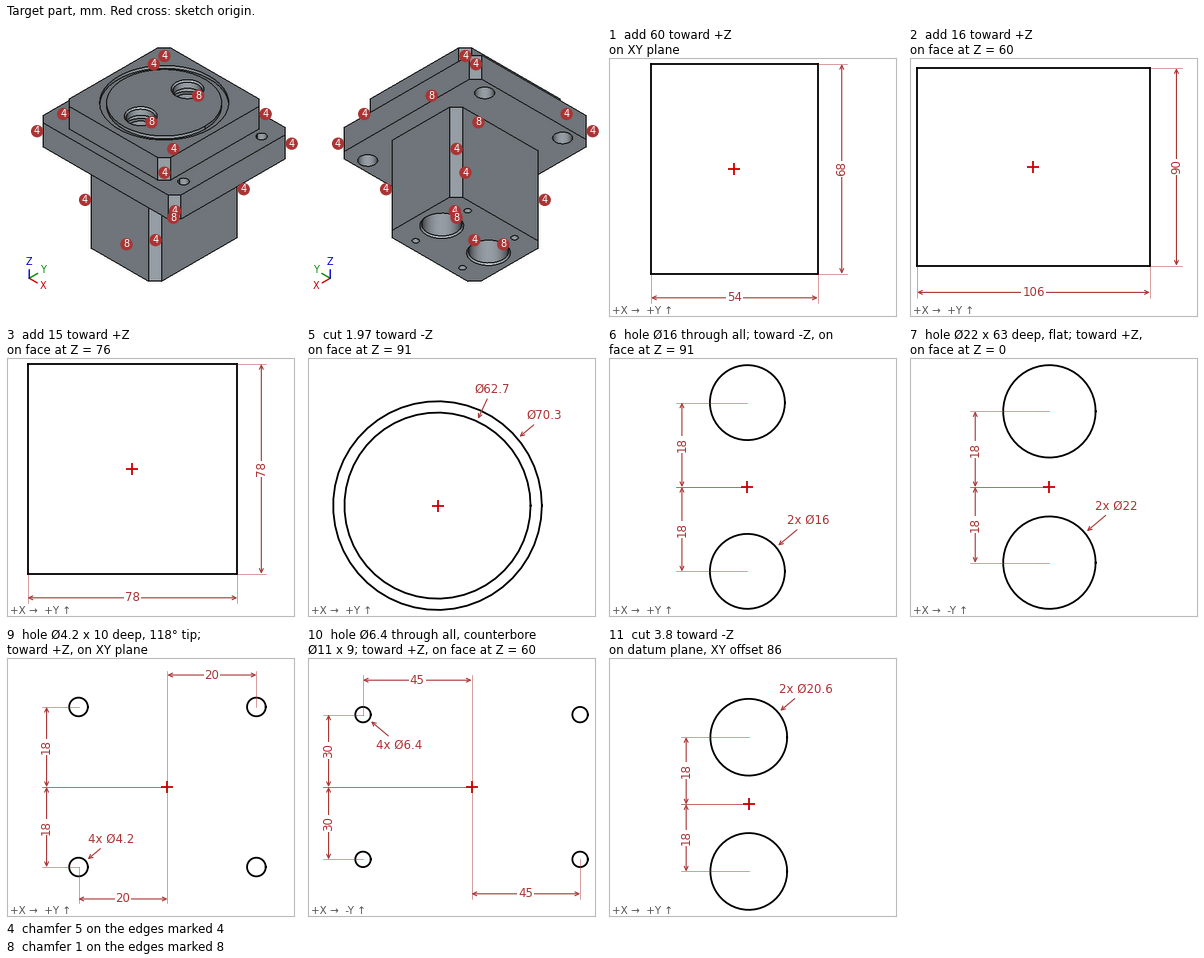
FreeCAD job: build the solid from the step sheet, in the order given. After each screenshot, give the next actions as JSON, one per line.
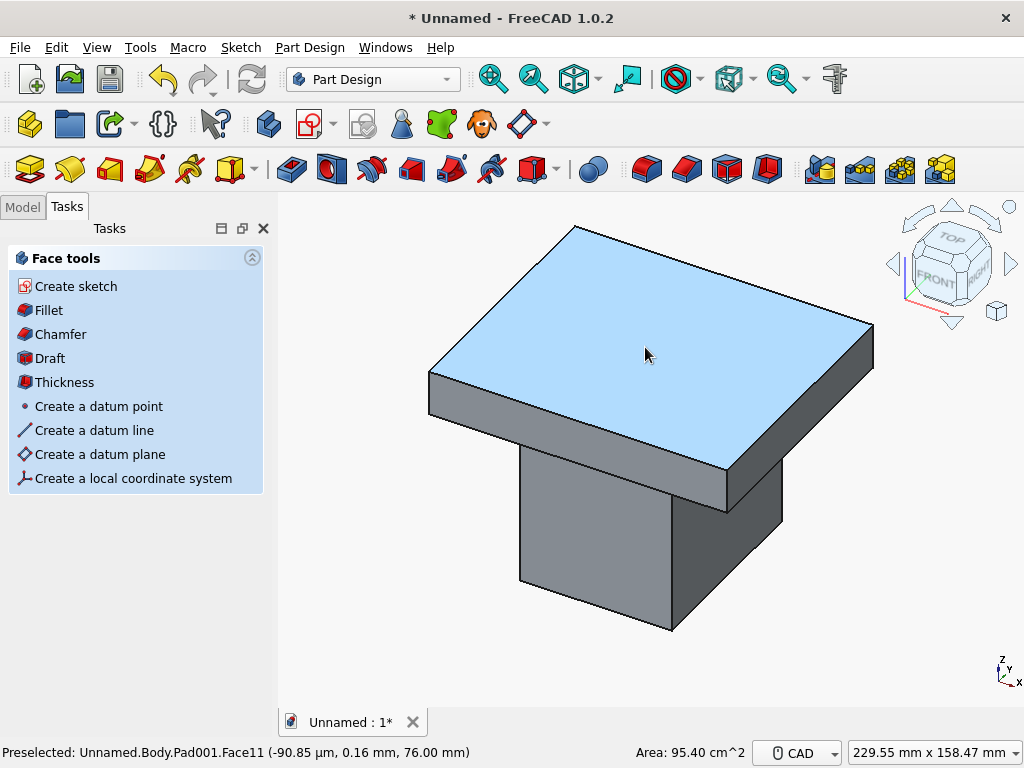
{"action": "left_click", "coordinate": [310, 124]}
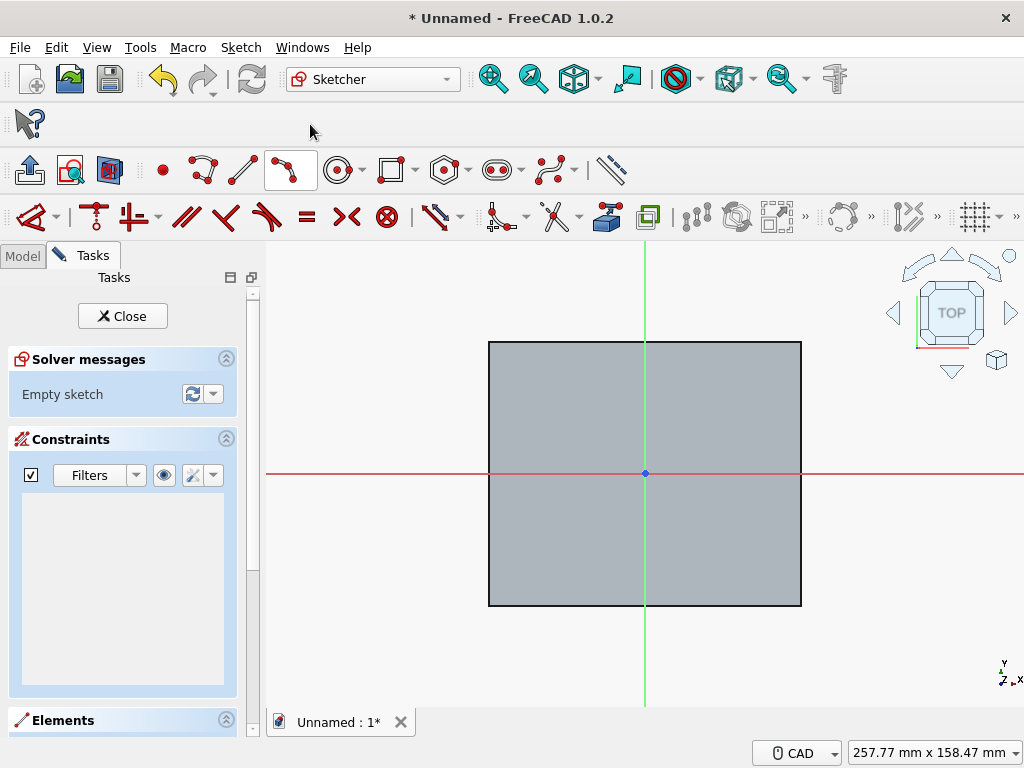
{"action": "key", "text": "g v"}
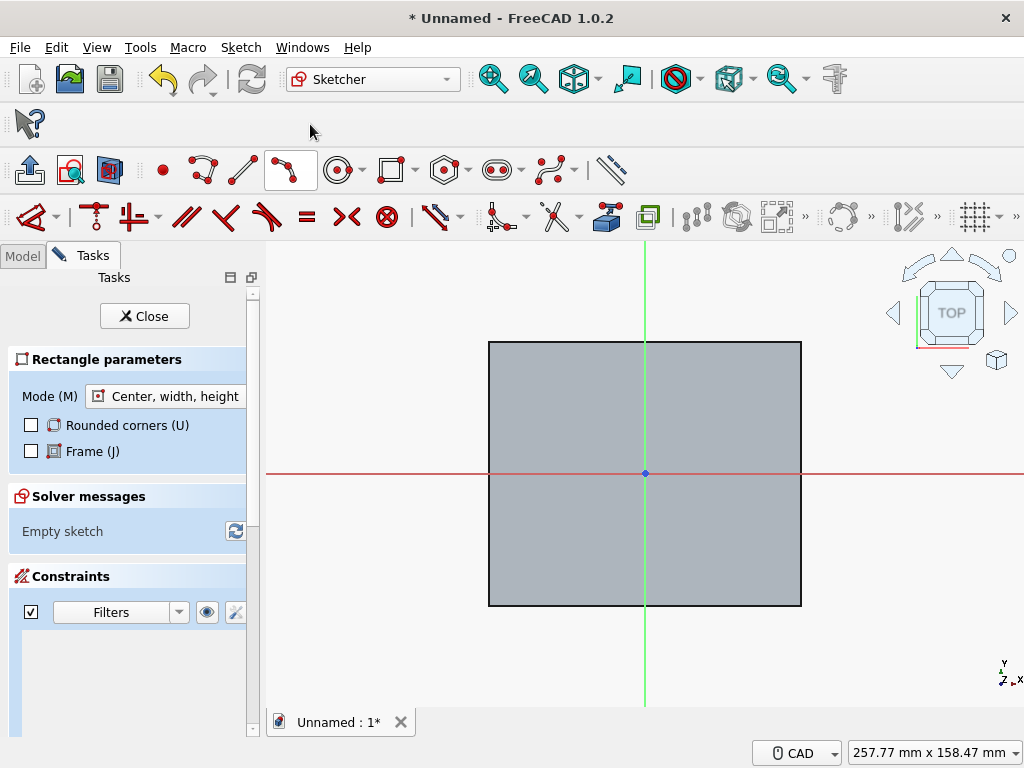
{"action": "left_click", "coordinate": [645, 474]}
{"action": "mouse_move", "coordinate": [760, 359]}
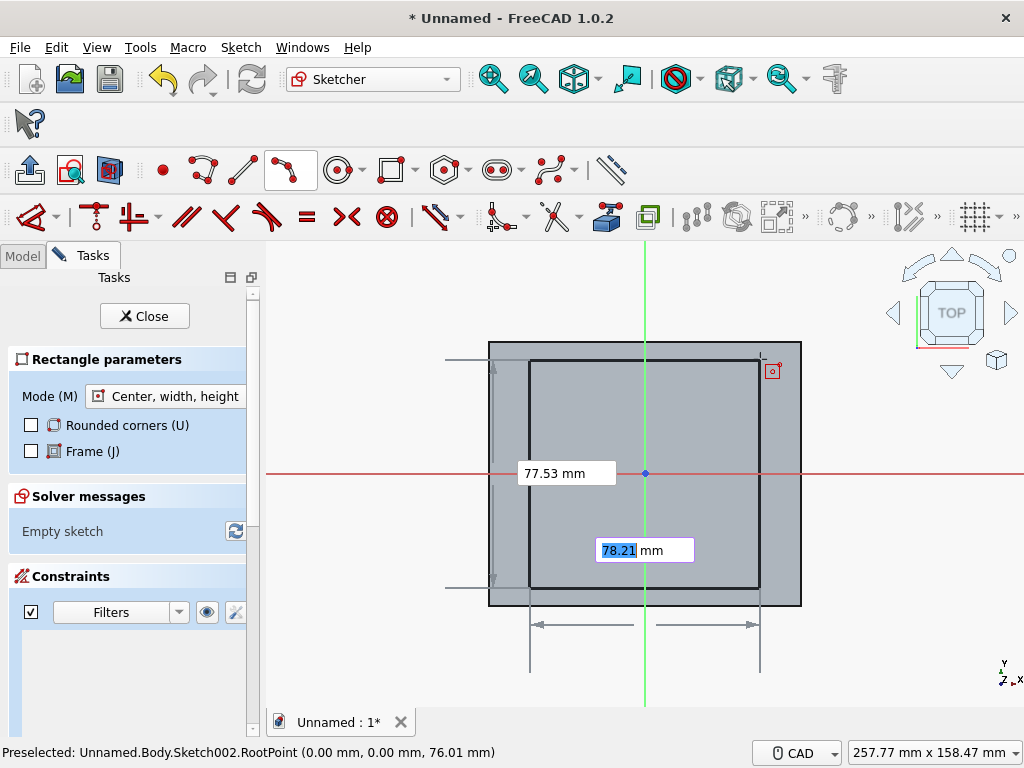
{"action": "type", "text": "78"}
{"action": "key", "text": "Tab"}
{"action": "type", "text": "78"}
{"action": "key", "text": "Return"}
{"action": "key", "text": "Escape"}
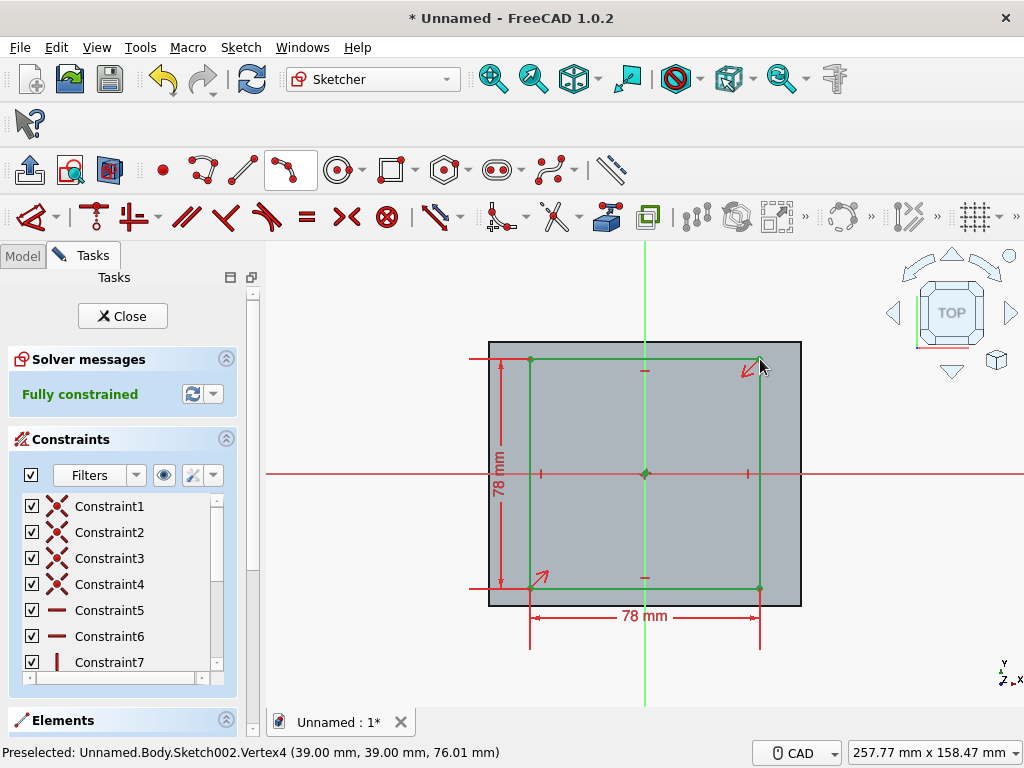
{"action": "left_click", "coordinate": [123, 316]}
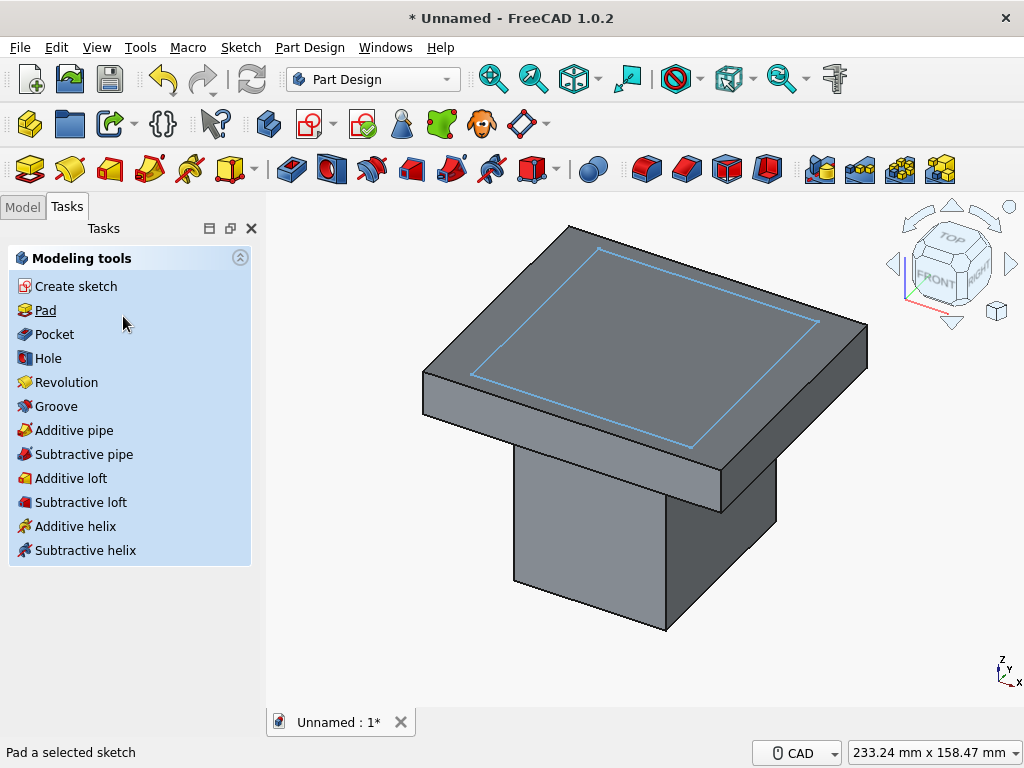
{"action": "left_click", "coordinate": [30, 170]}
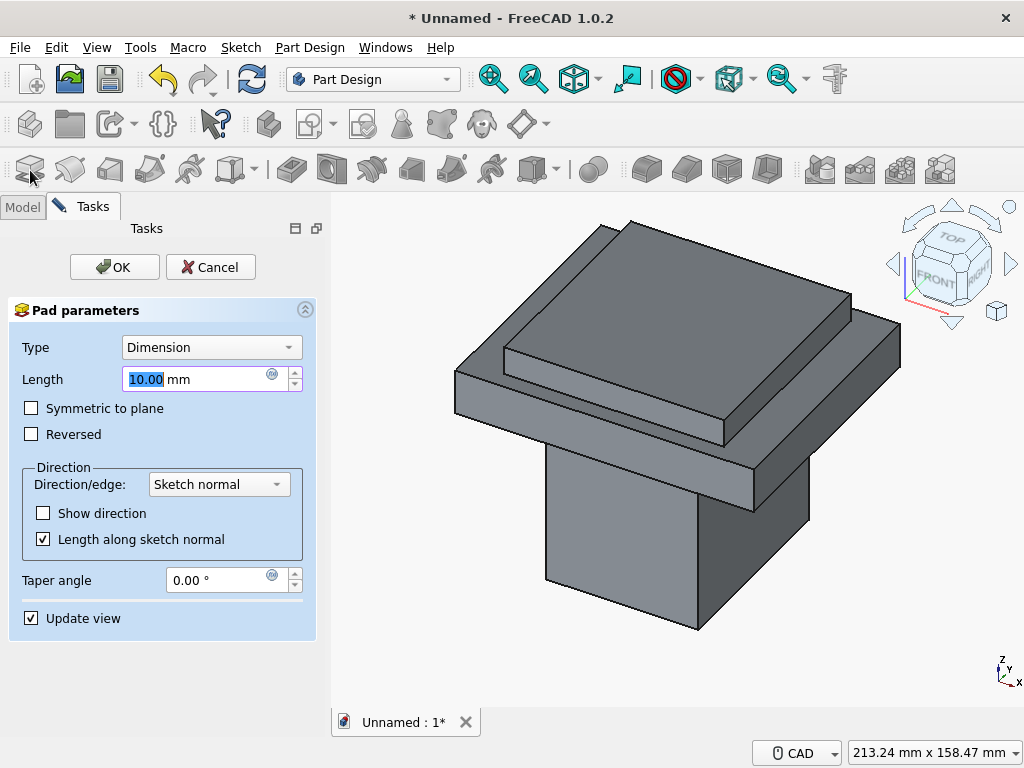
{"action": "type", "text": "15"}
{"action": "key", "text": "Tab"}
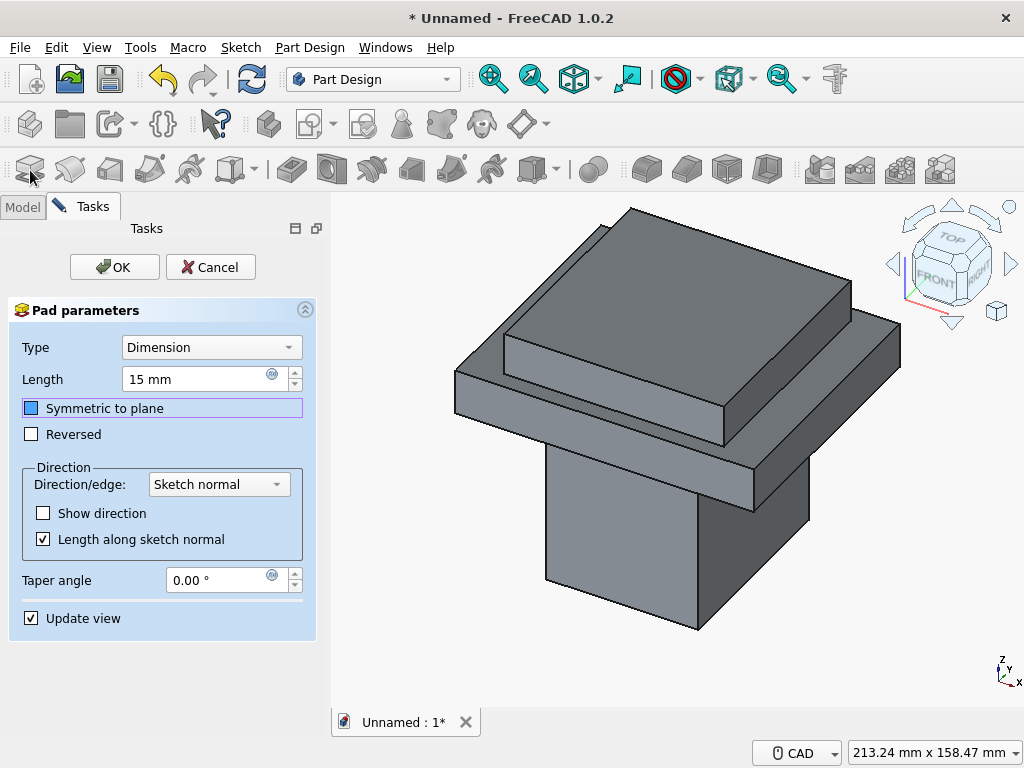
{"action": "left_click", "coordinate": [115, 267]}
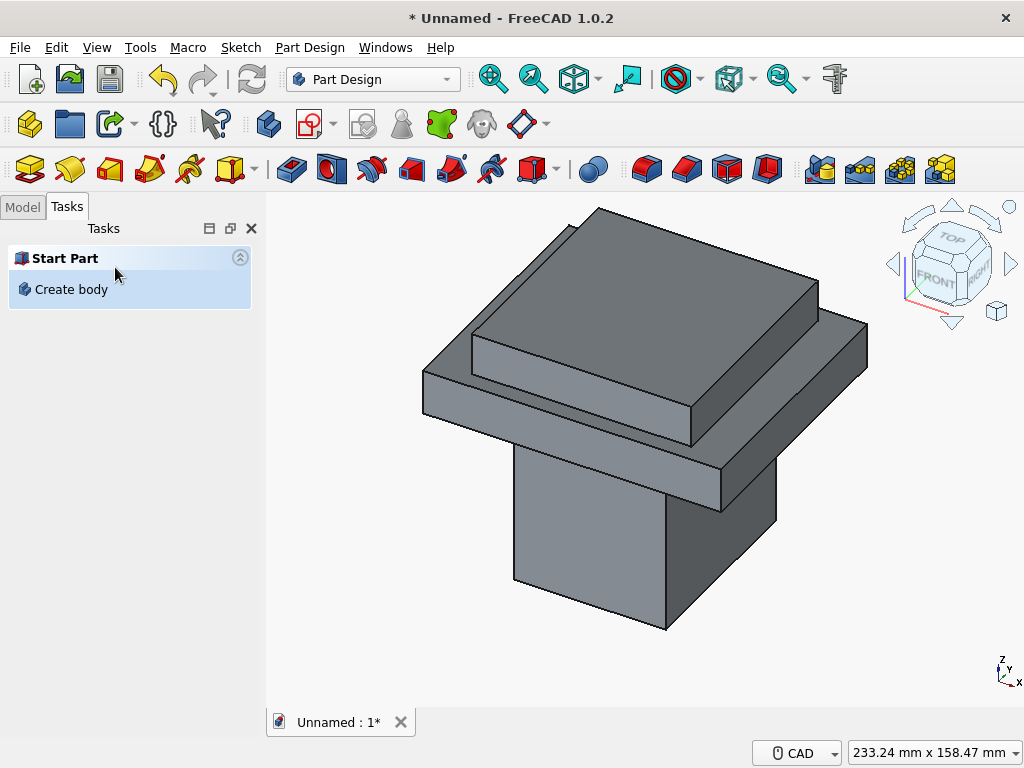
{"action": "key", "text": "v f"}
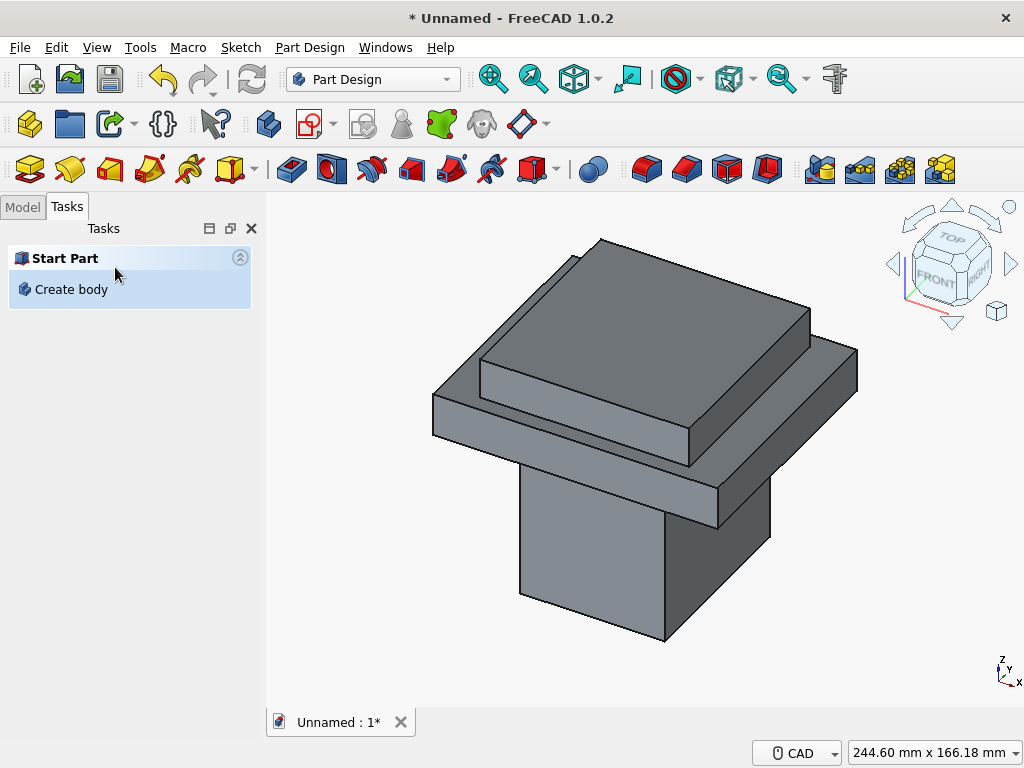
{"action": "left_click", "coordinate": [718, 508]}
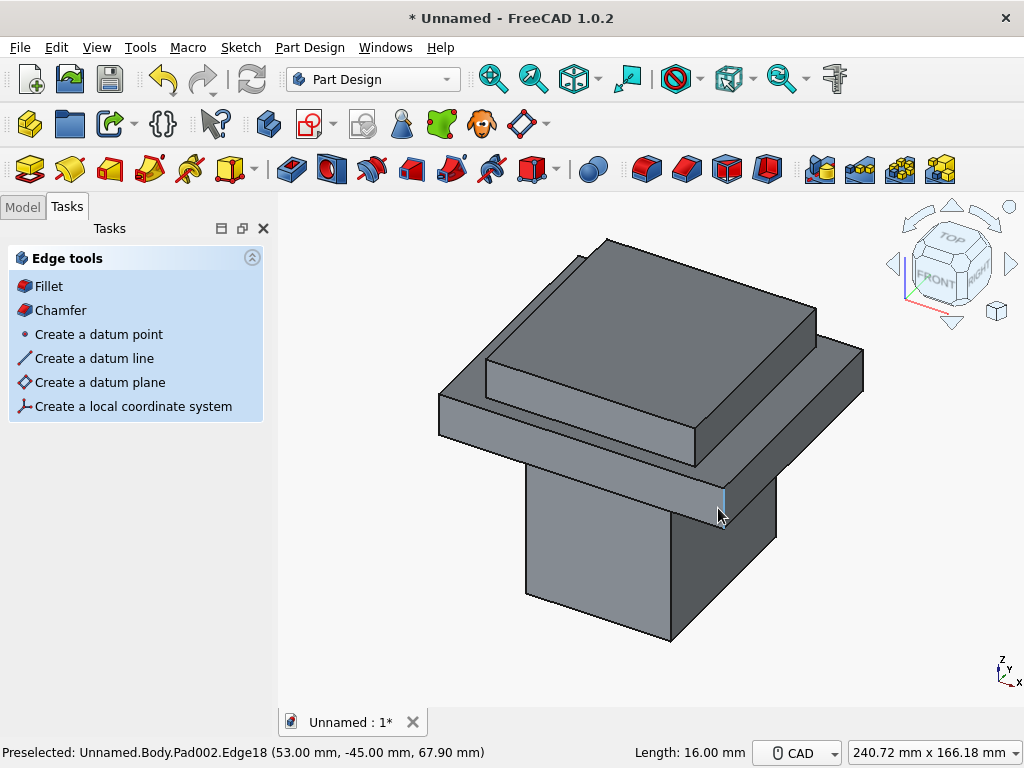
{"action": "left_click", "coordinate": [695, 447], "text": "ctrl"}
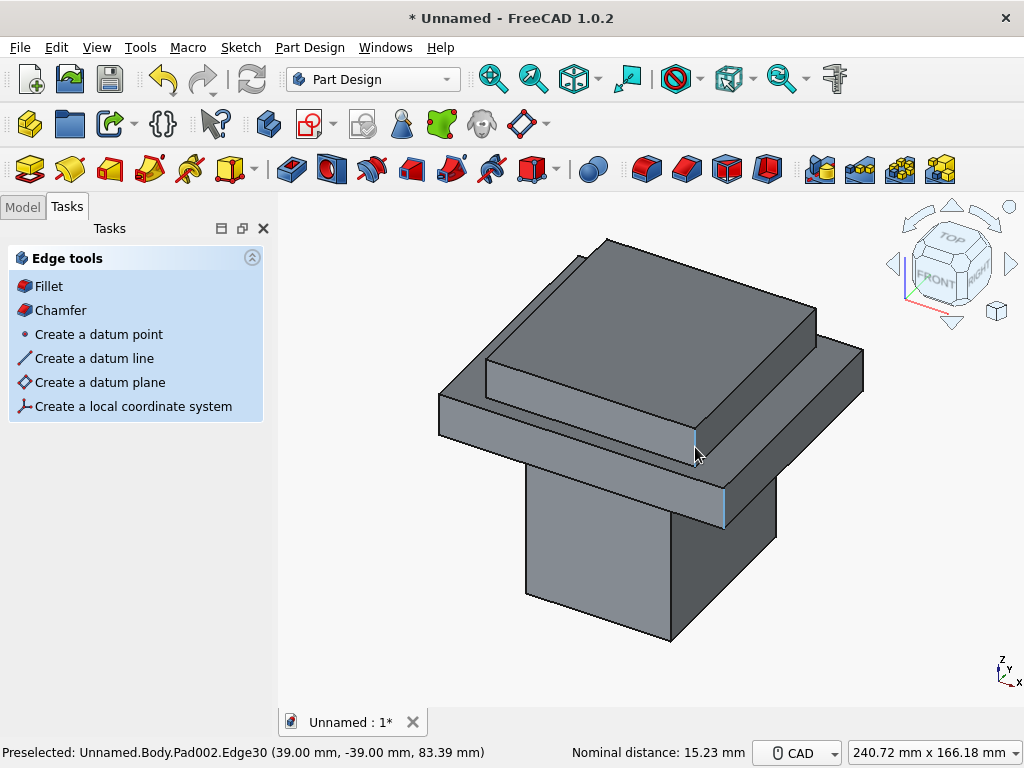
{"action": "left_click", "coordinate": [671, 564], "text": "ctrl"}